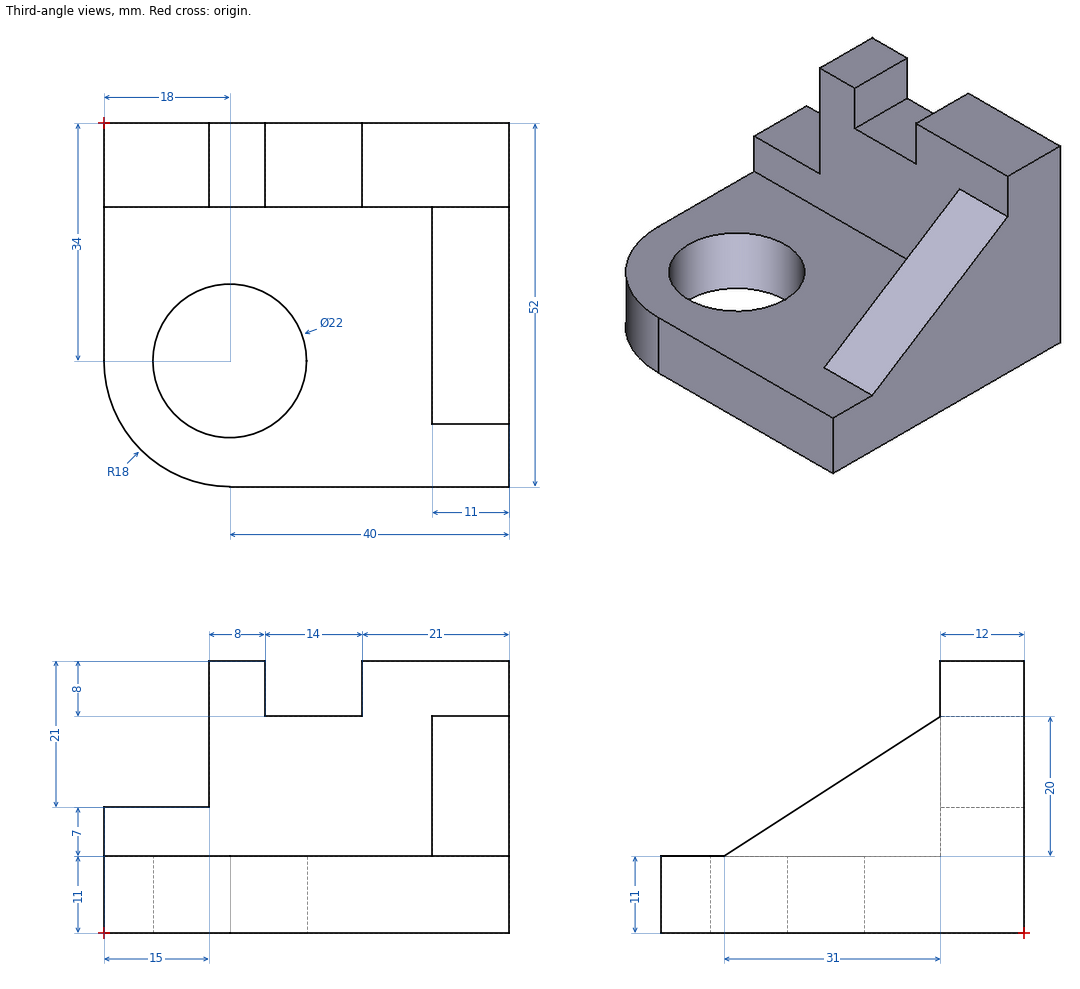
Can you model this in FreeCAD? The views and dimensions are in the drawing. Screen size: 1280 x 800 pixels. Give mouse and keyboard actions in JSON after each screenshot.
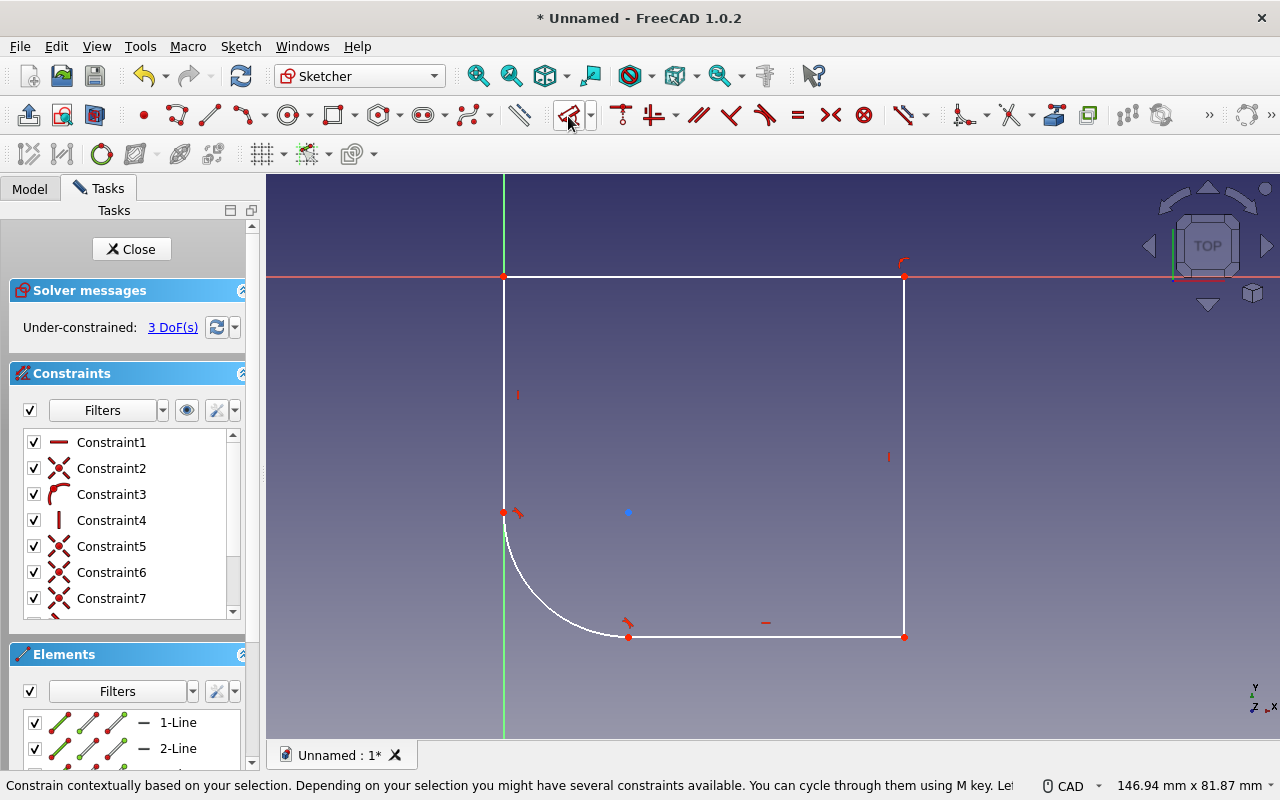
{"action": "left_click", "coordinate": [518, 569]}
{"action": "left_click", "coordinate": [490, 584]}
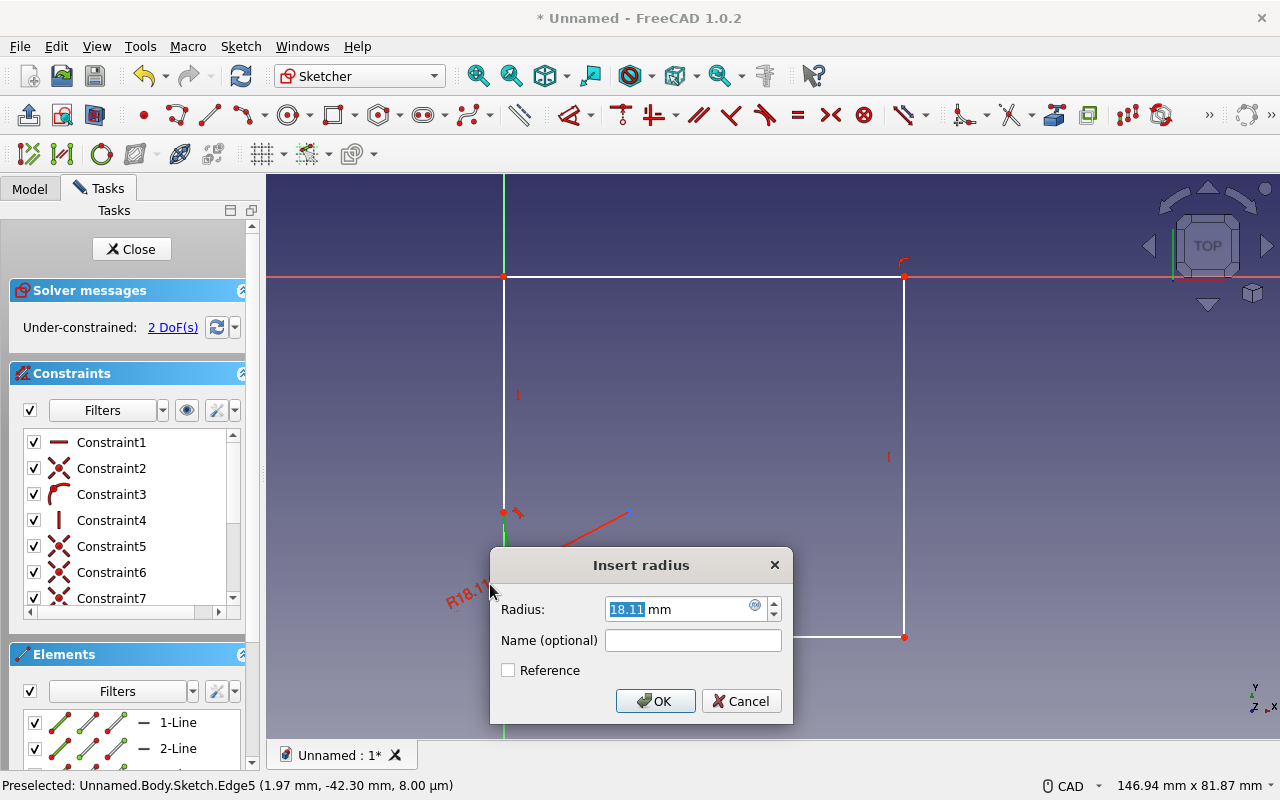
{"action": "type", "text": "18"}
{"action": "key", "text": "Return"}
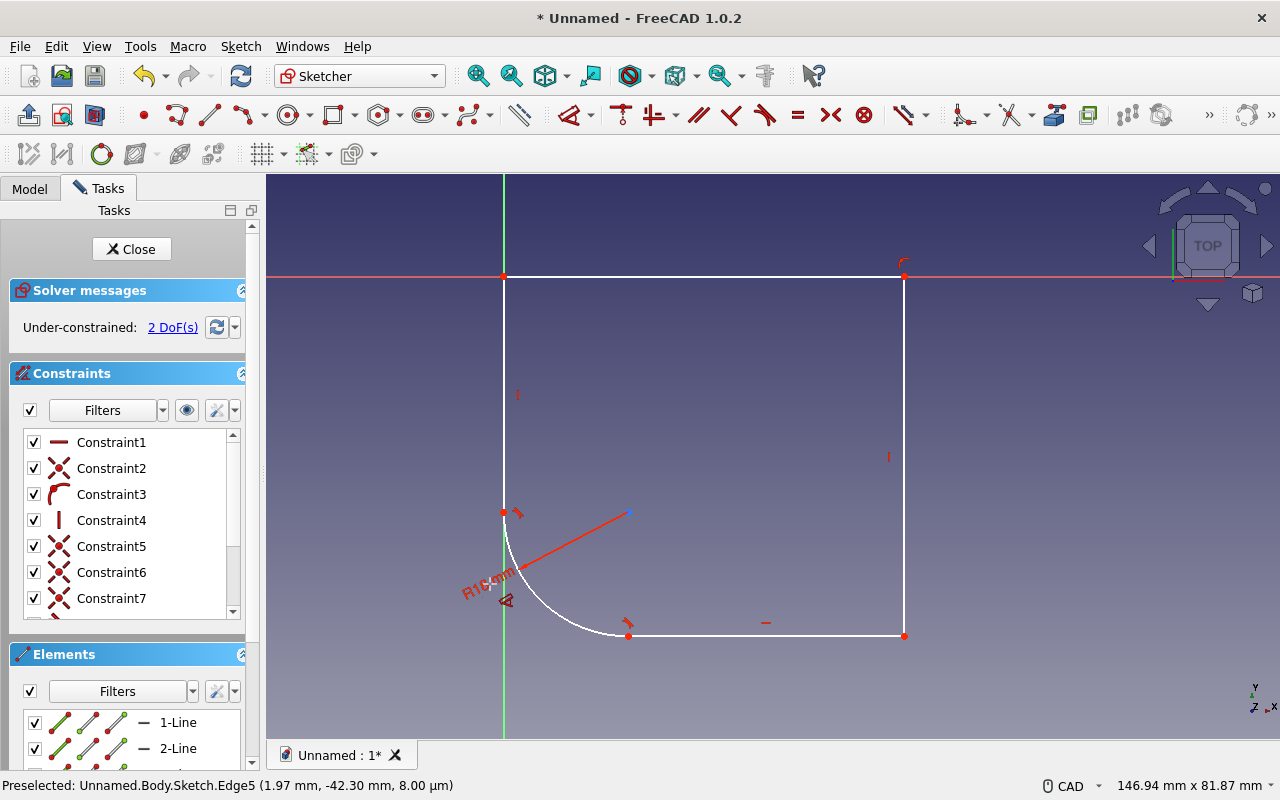
{"action": "left_click", "coordinate": [711, 636]}
{"action": "left_click", "coordinate": [766, 670]}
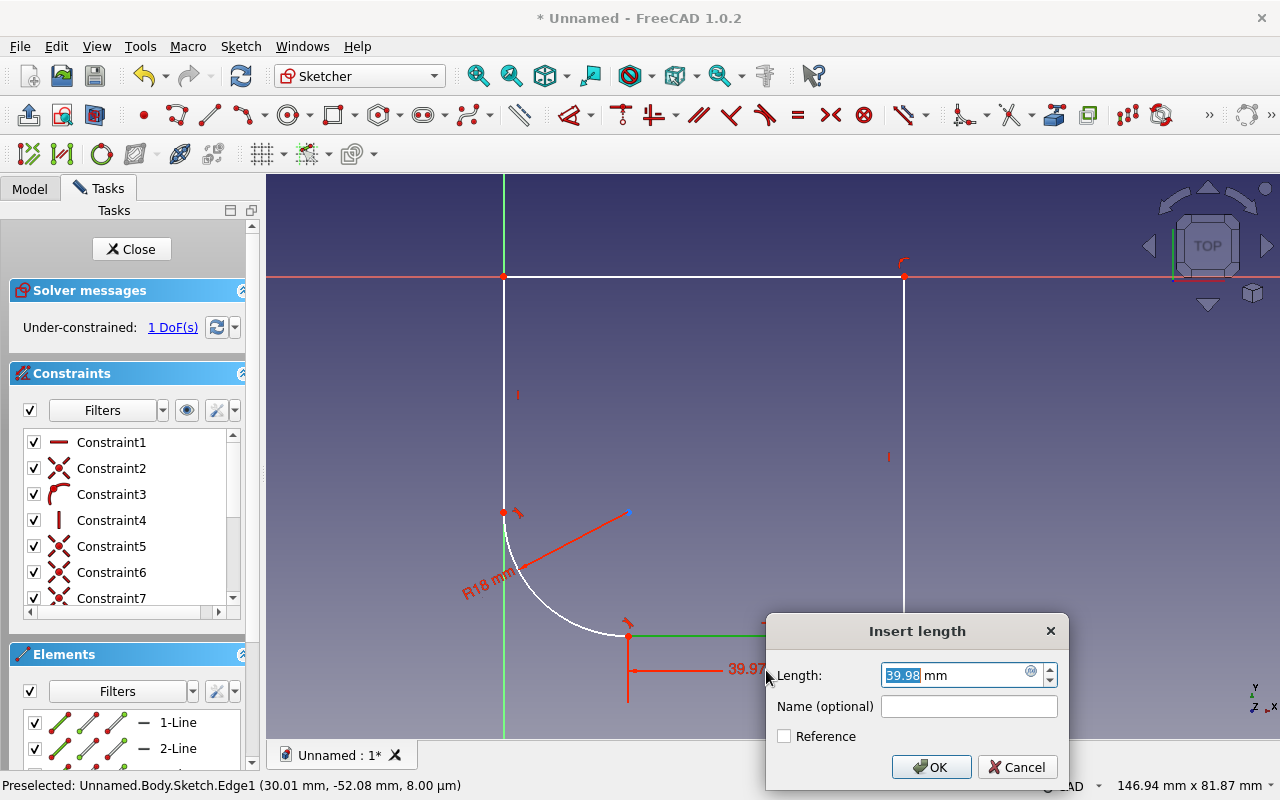
{"action": "type", "text": "40"}
{"action": "key", "text": "Return"}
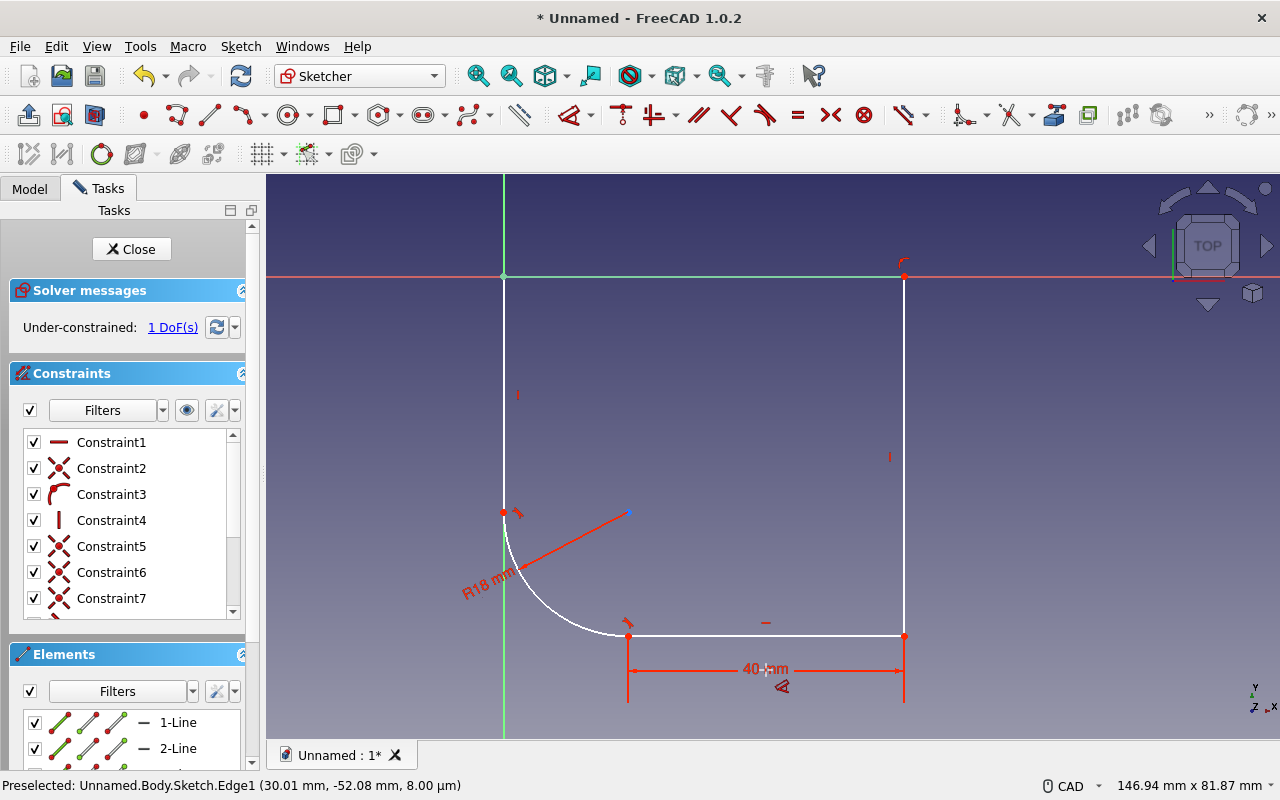
{"action": "left_click", "coordinate": [904, 528]}
{"action": "left_click", "coordinate": [938, 457]}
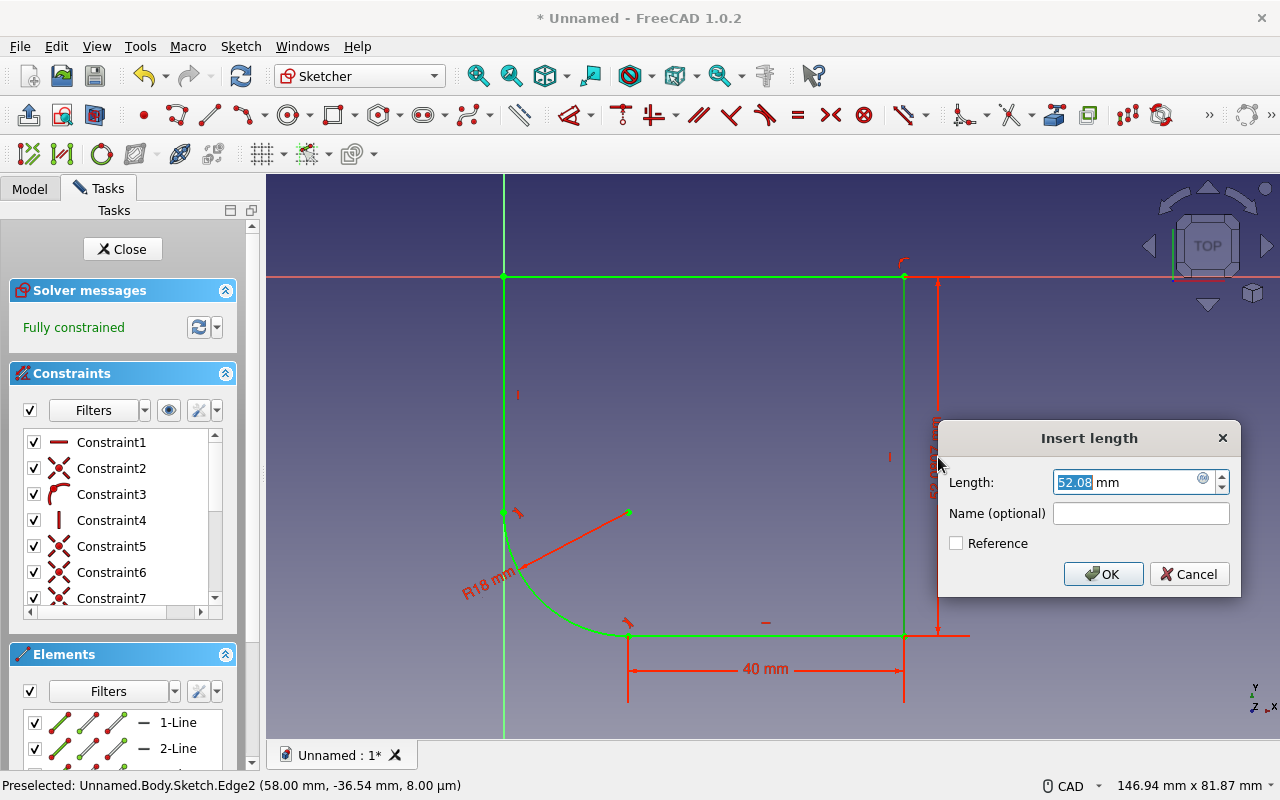
{"action": "type", "text": "52"}
{"action": "key", "text": "Return"}
{"action": "key", "text": "Escape"}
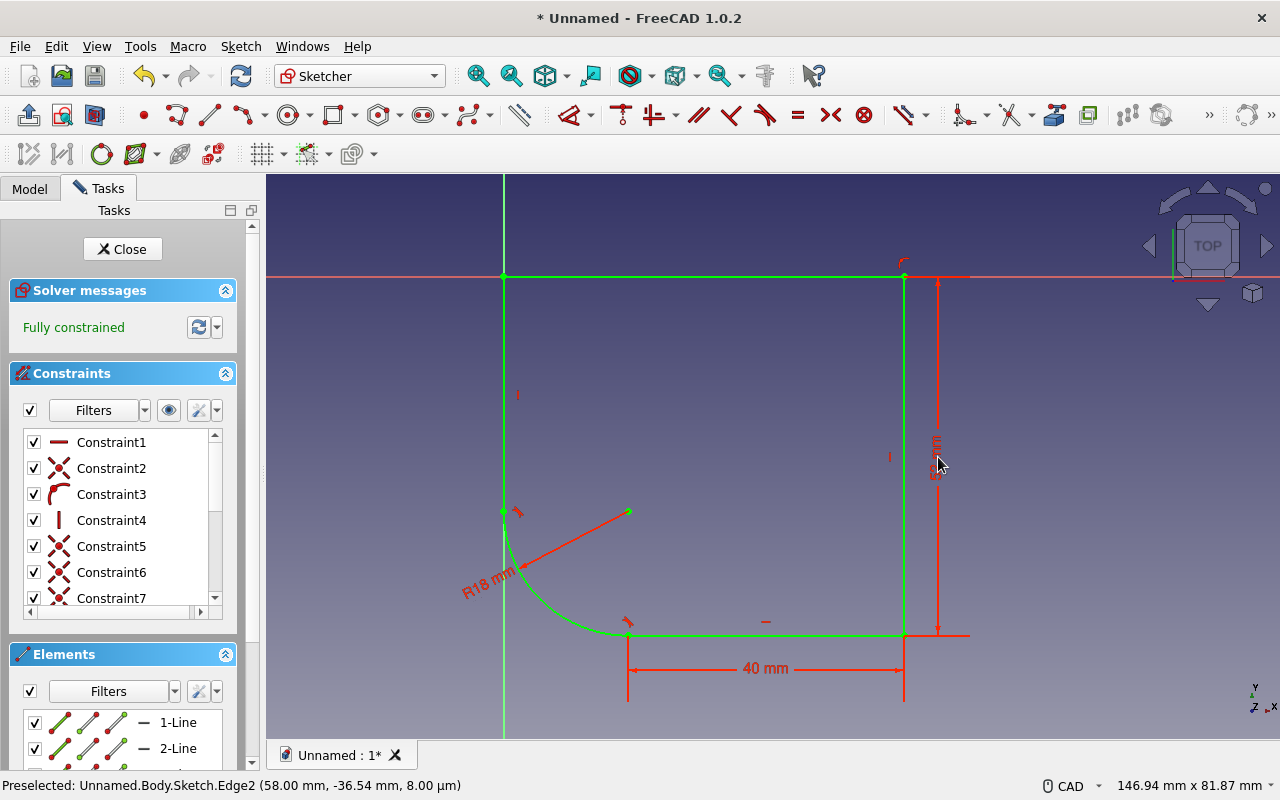
{"action": "left_click", "coordinate": [123, 249]}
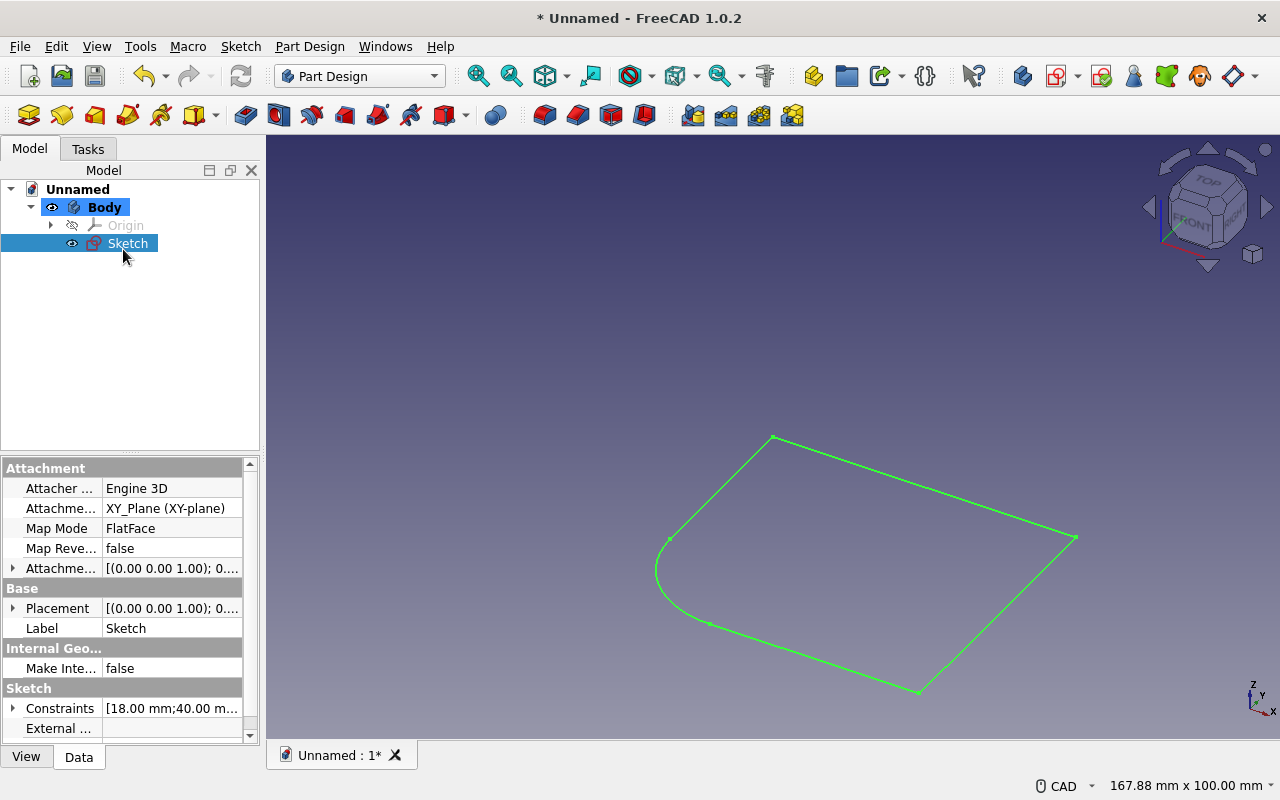
{"action": "left_click", "coordinate": [29, 116]}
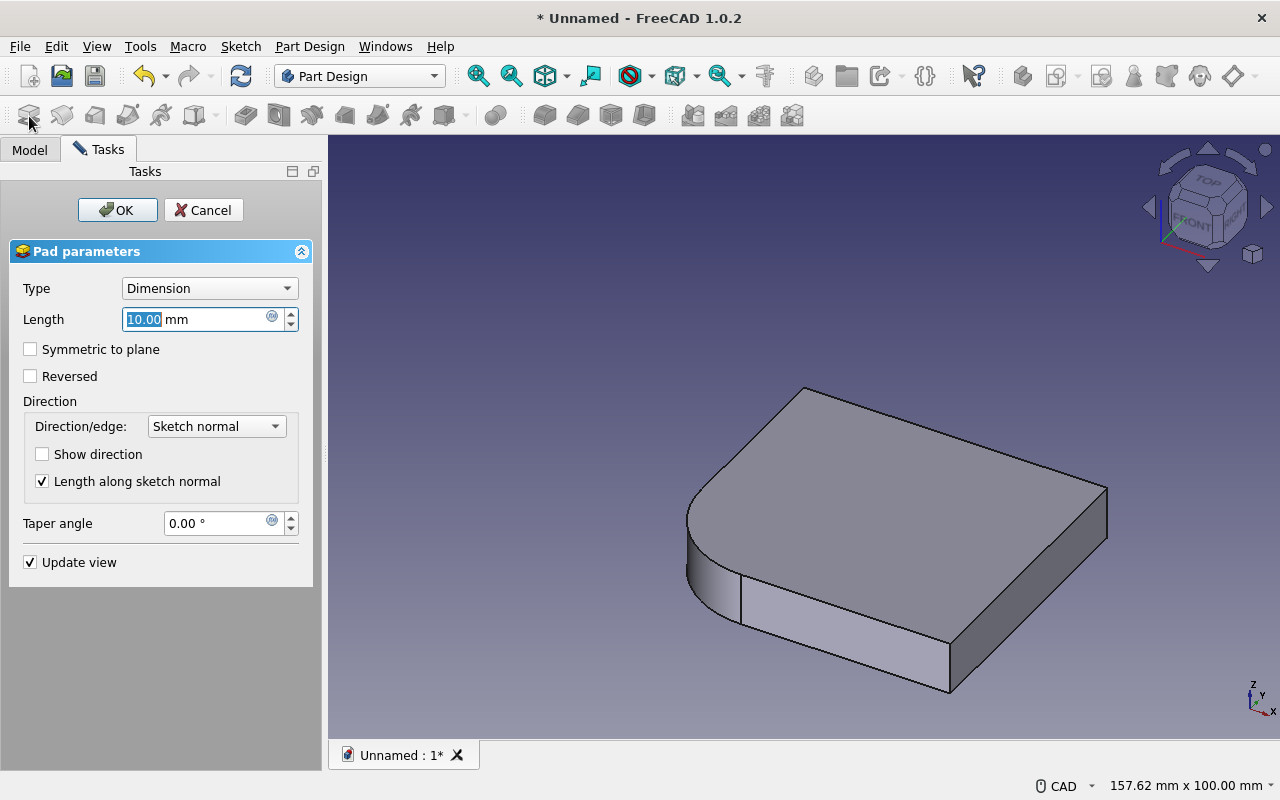
{"action": "type", "text": "11"}
{"action": "key", "text": "Tab"}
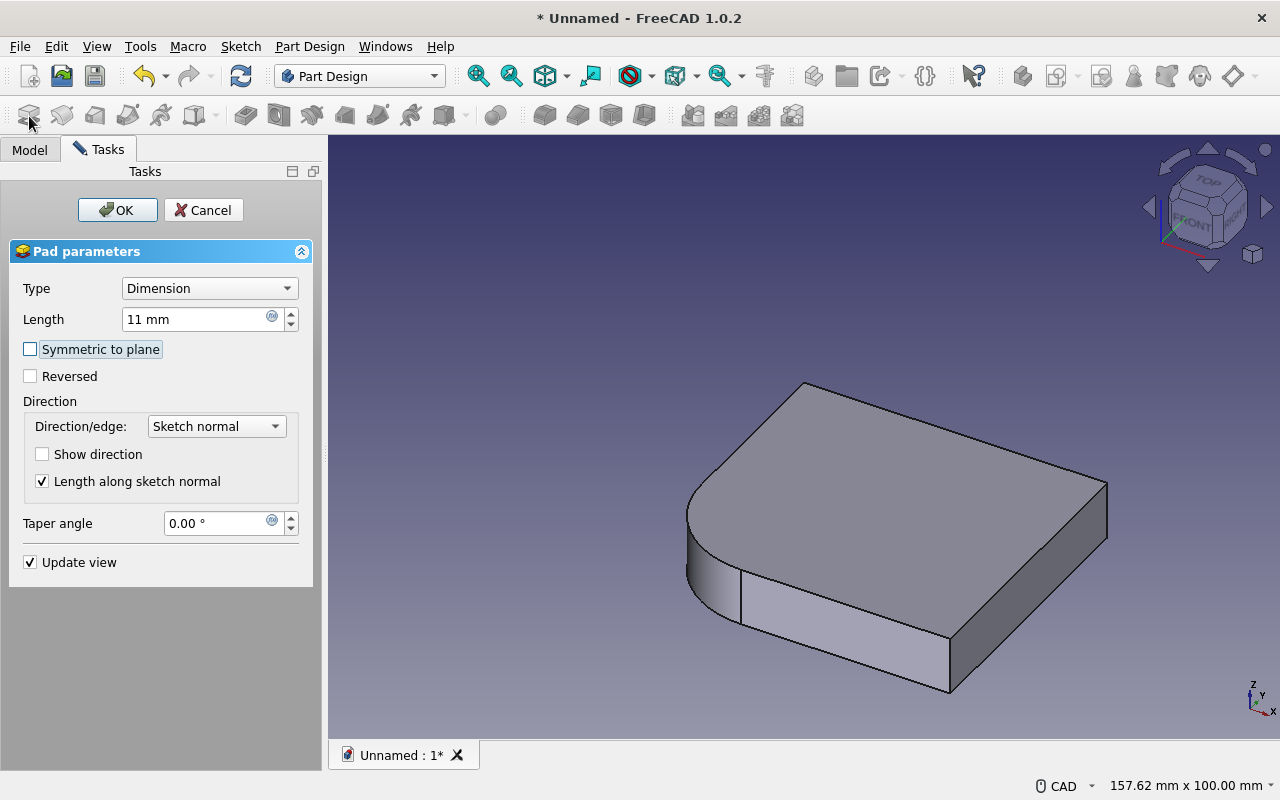
{"action": "left_click", "coordinate": [118, 210]}